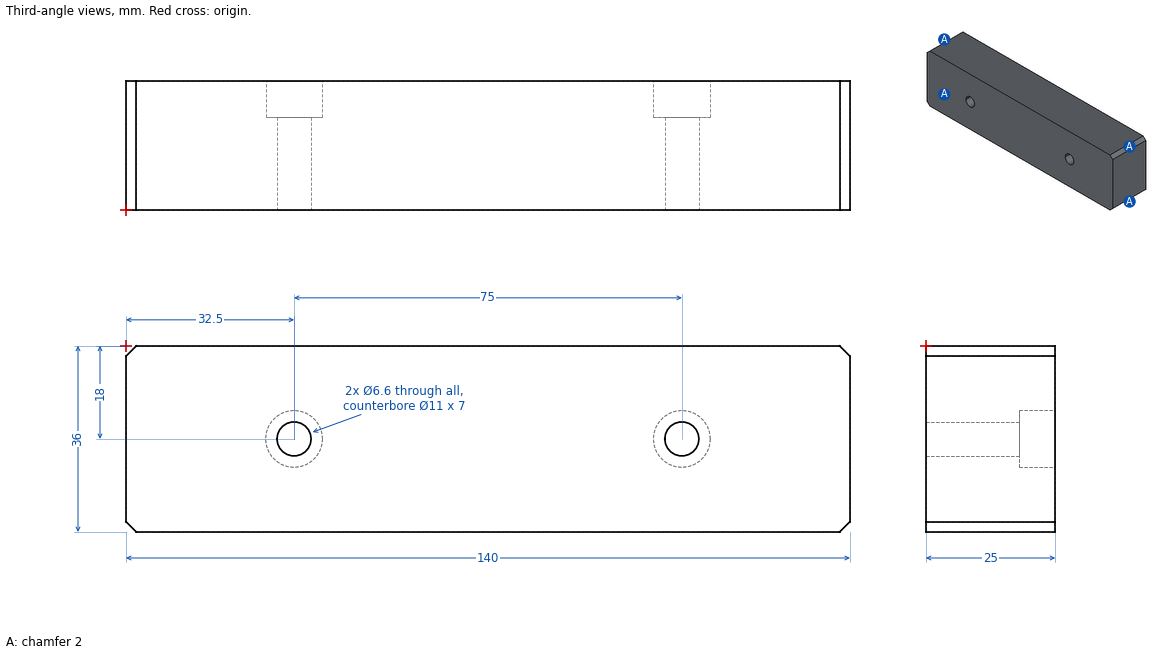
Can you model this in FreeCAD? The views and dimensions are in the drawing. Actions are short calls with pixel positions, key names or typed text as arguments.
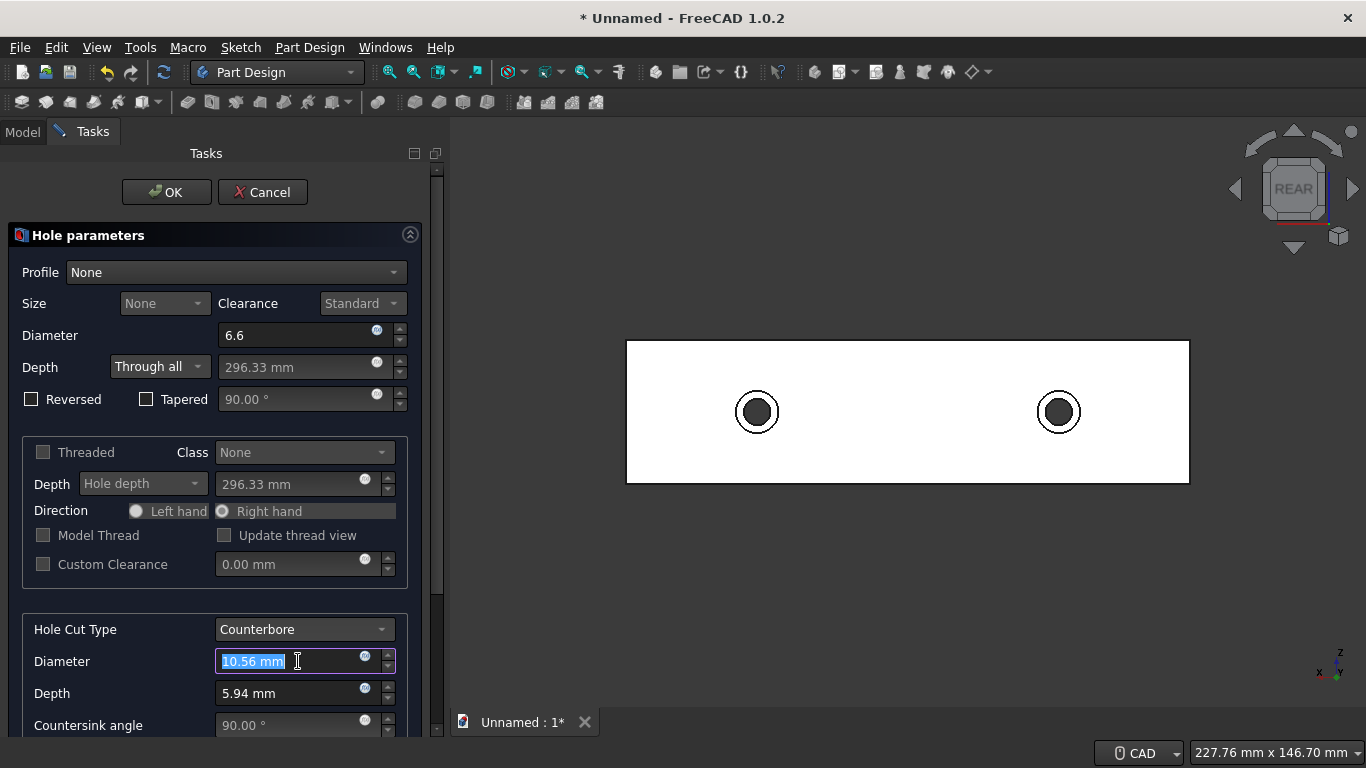
text(11)
key(Tab)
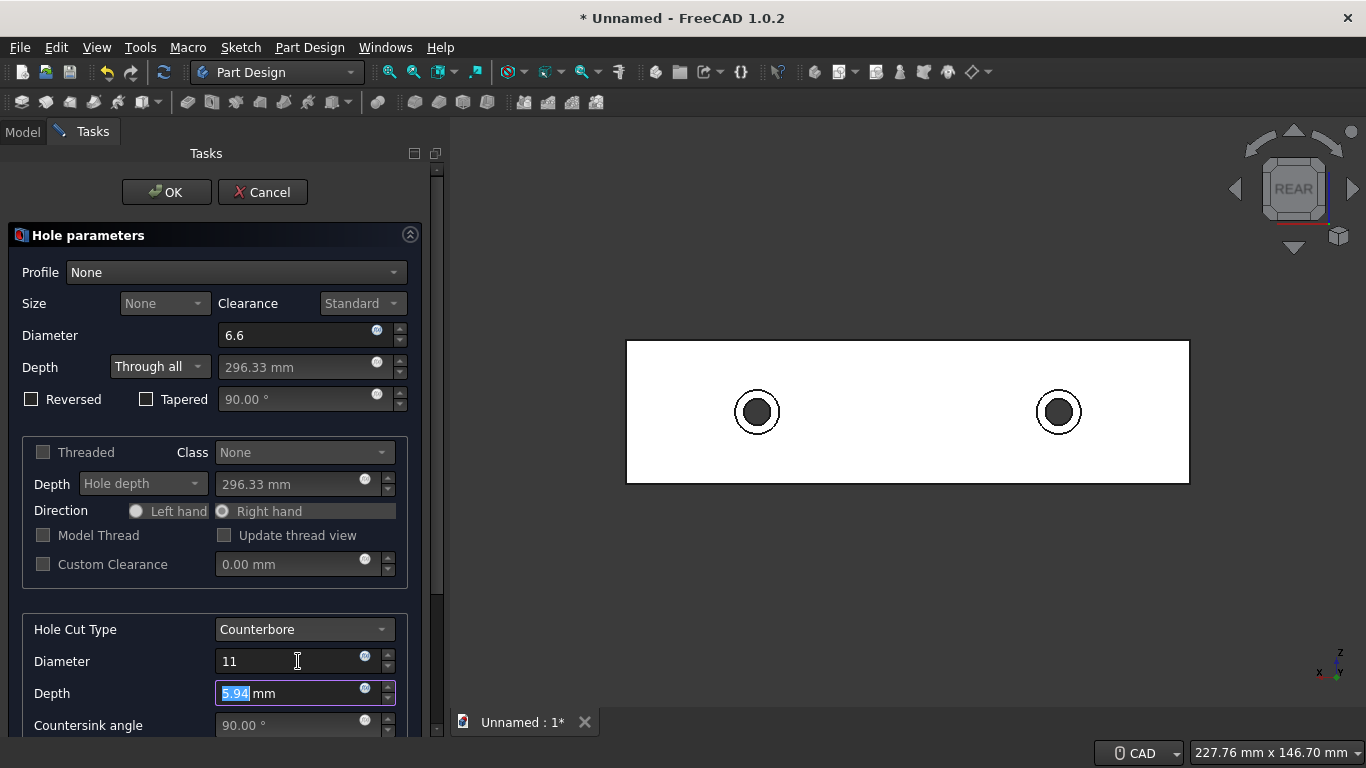
text(7)
key(Tab)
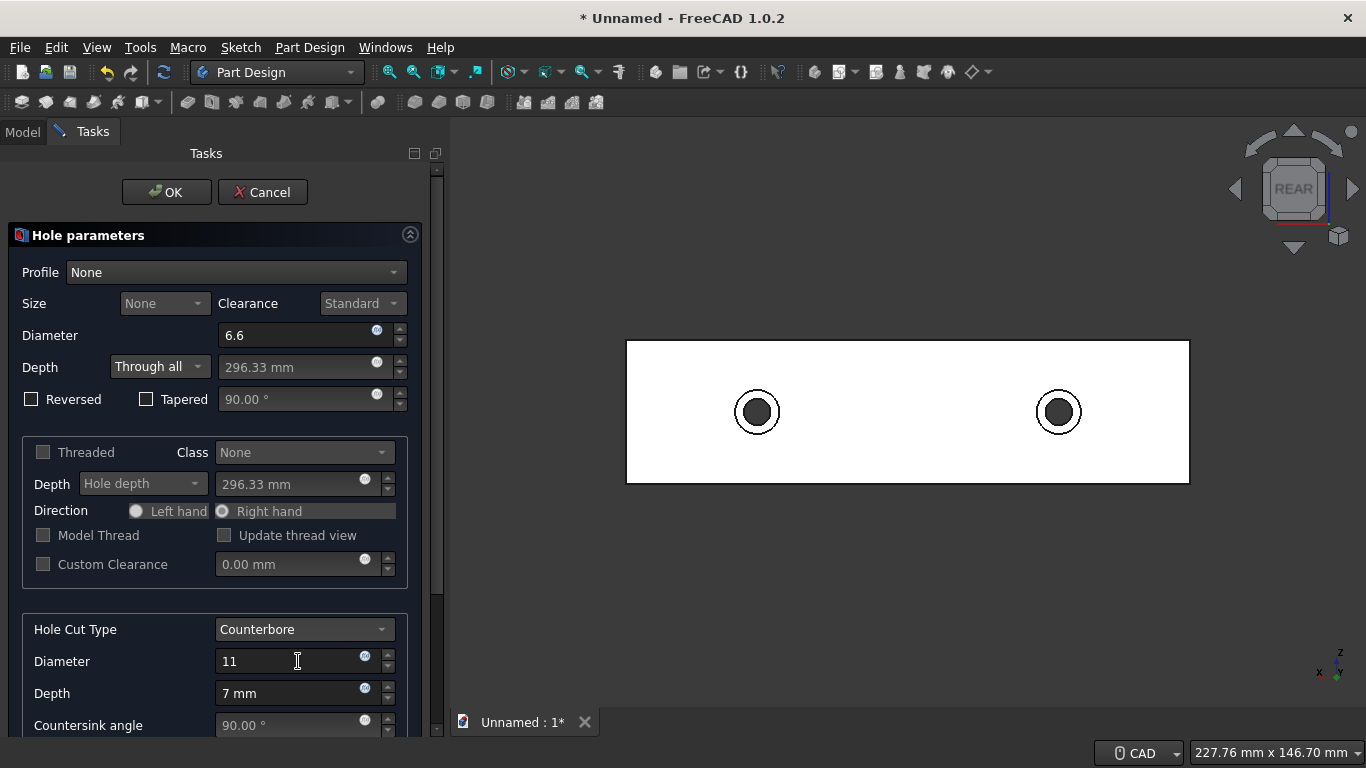
click(167, 192)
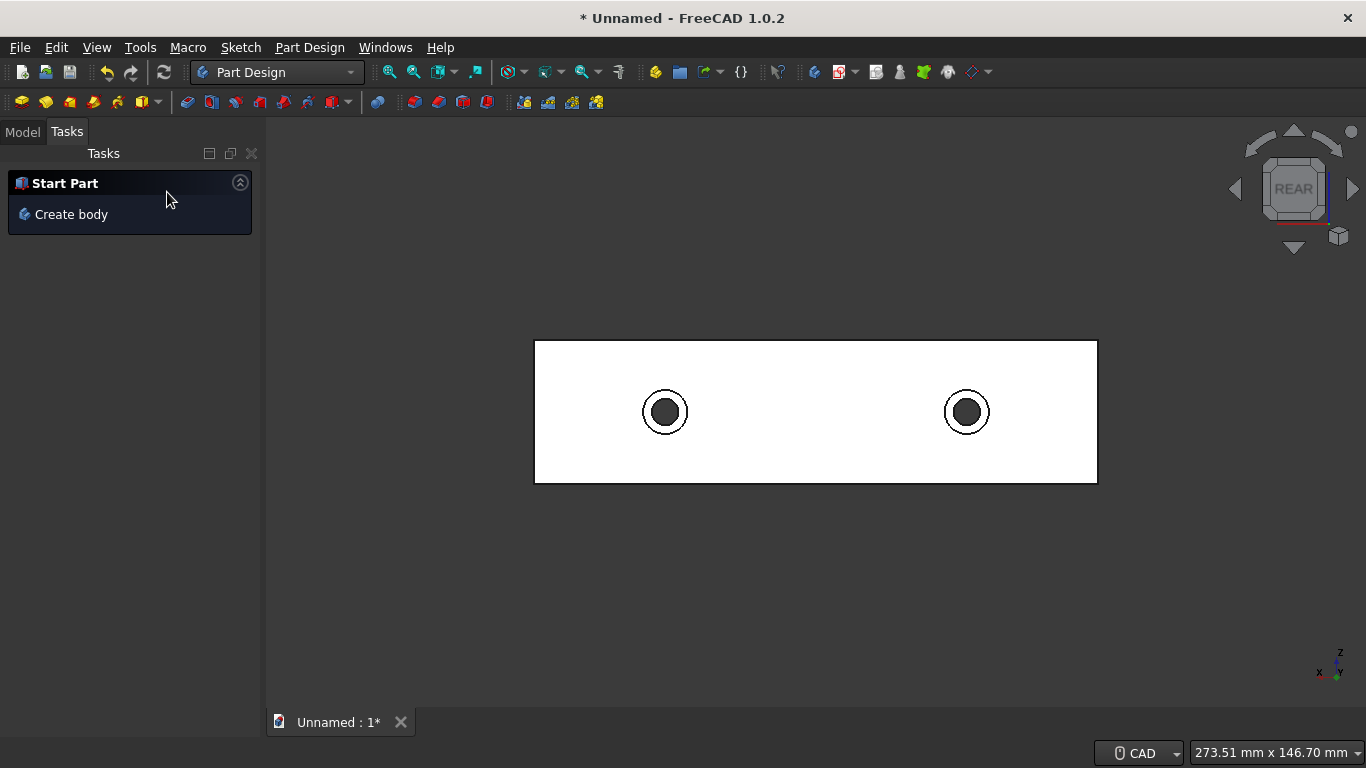
key(0)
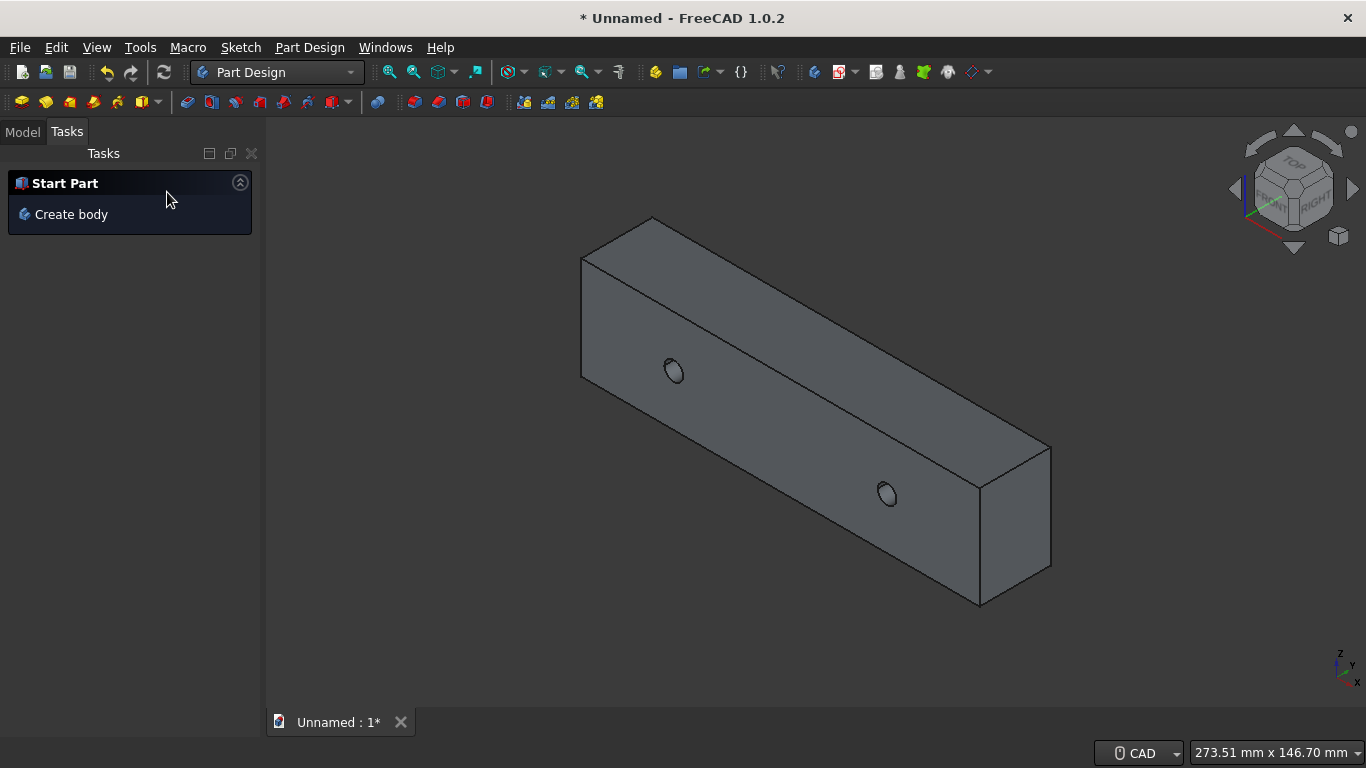
click(1015, 467)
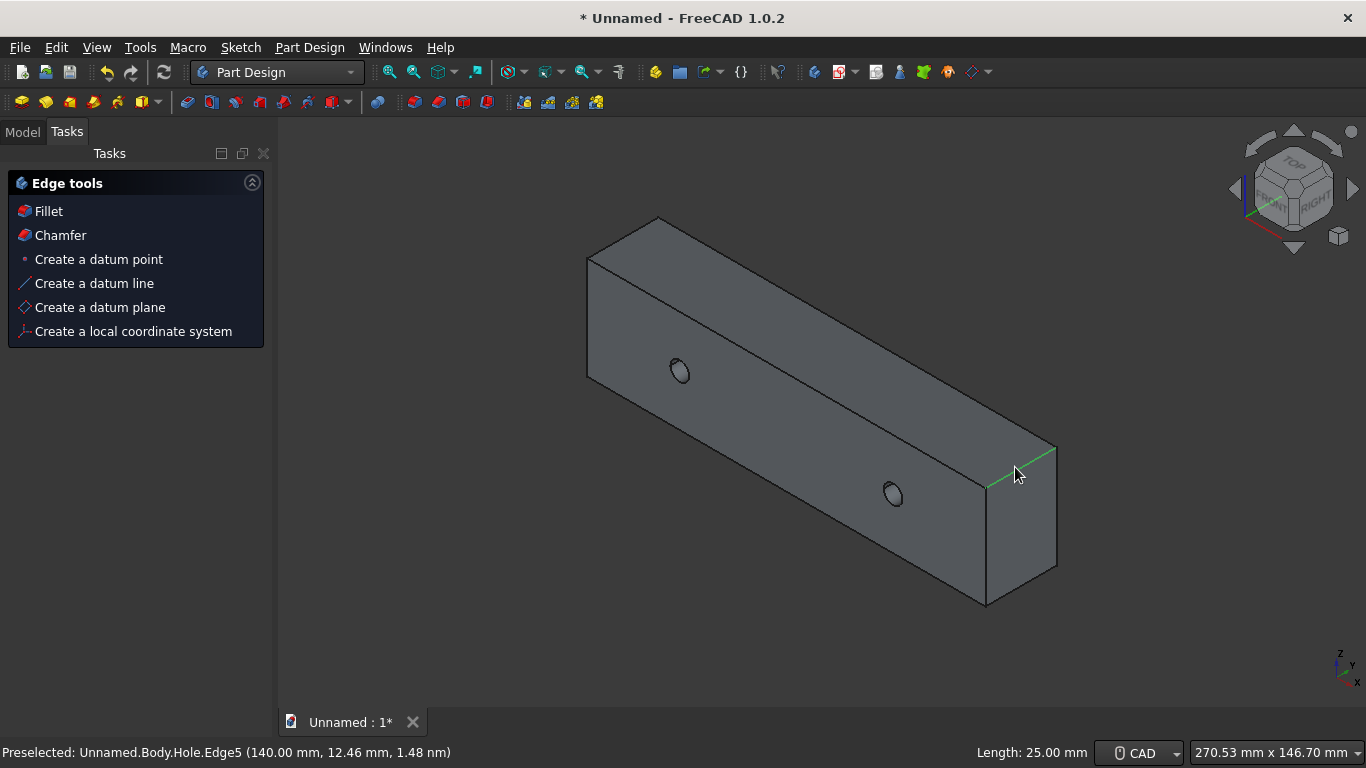
key(2)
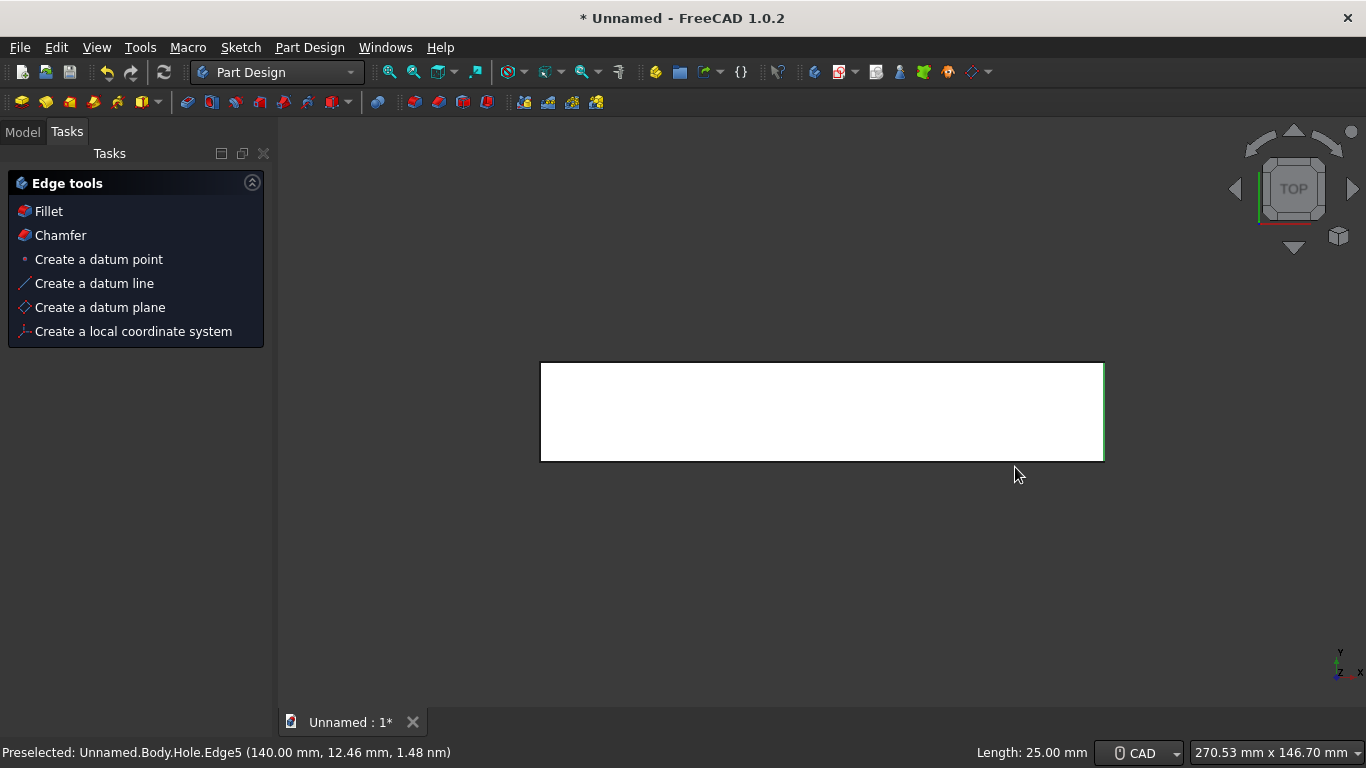
click(540, 421, ctrl)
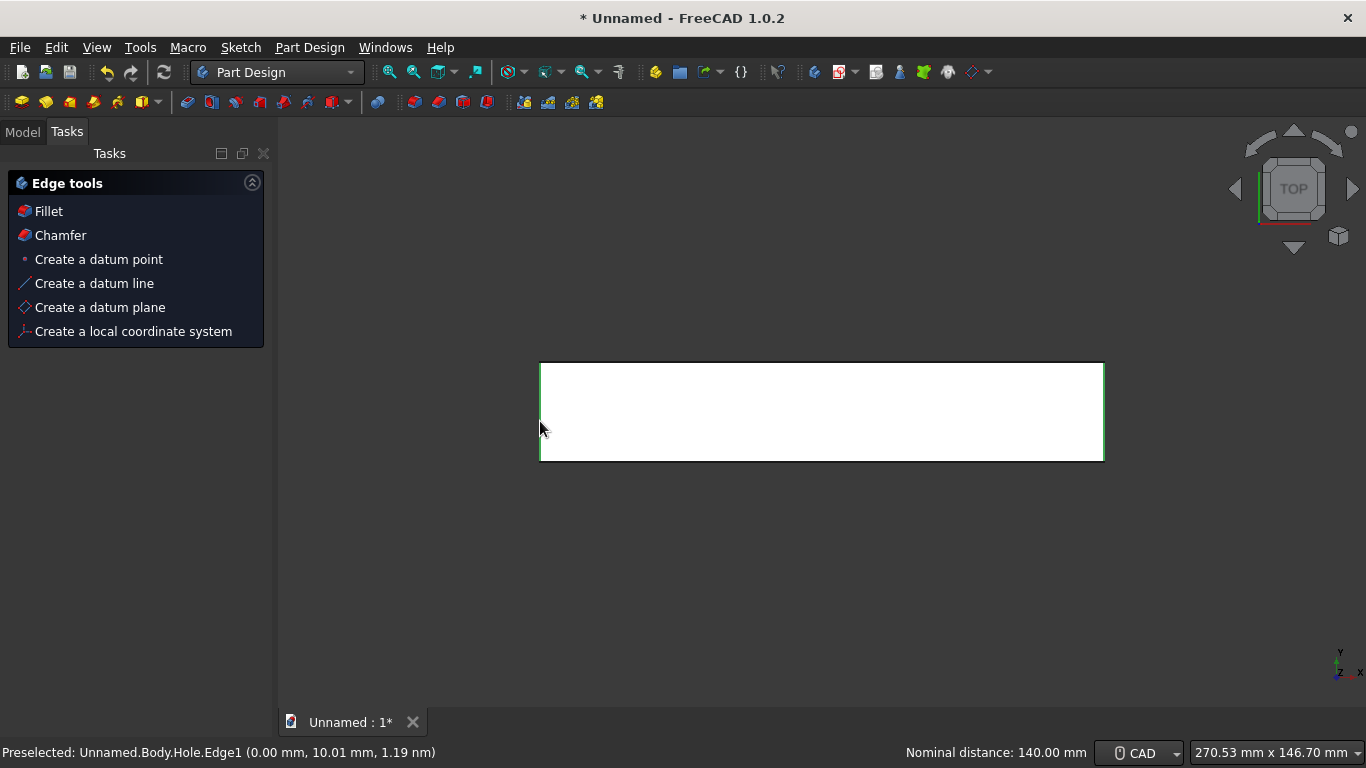
key(1)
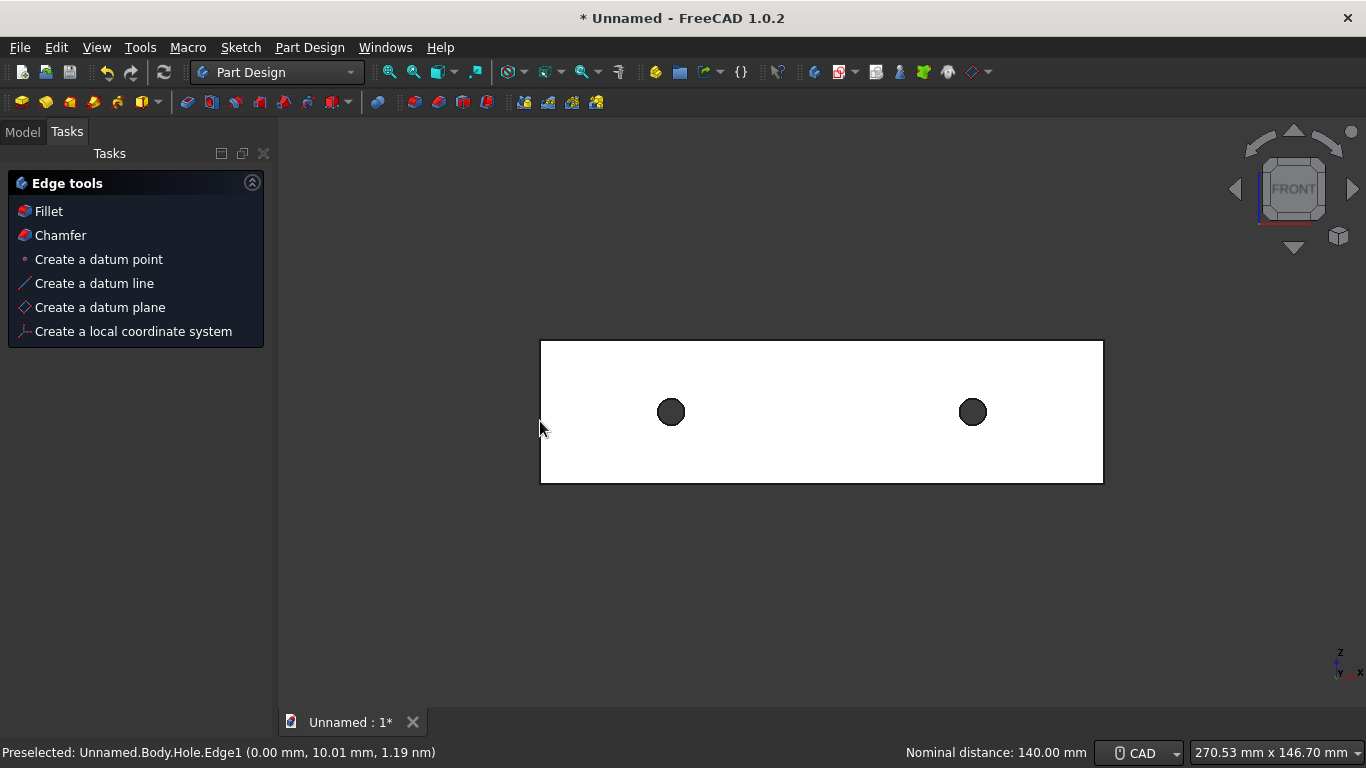
key(3)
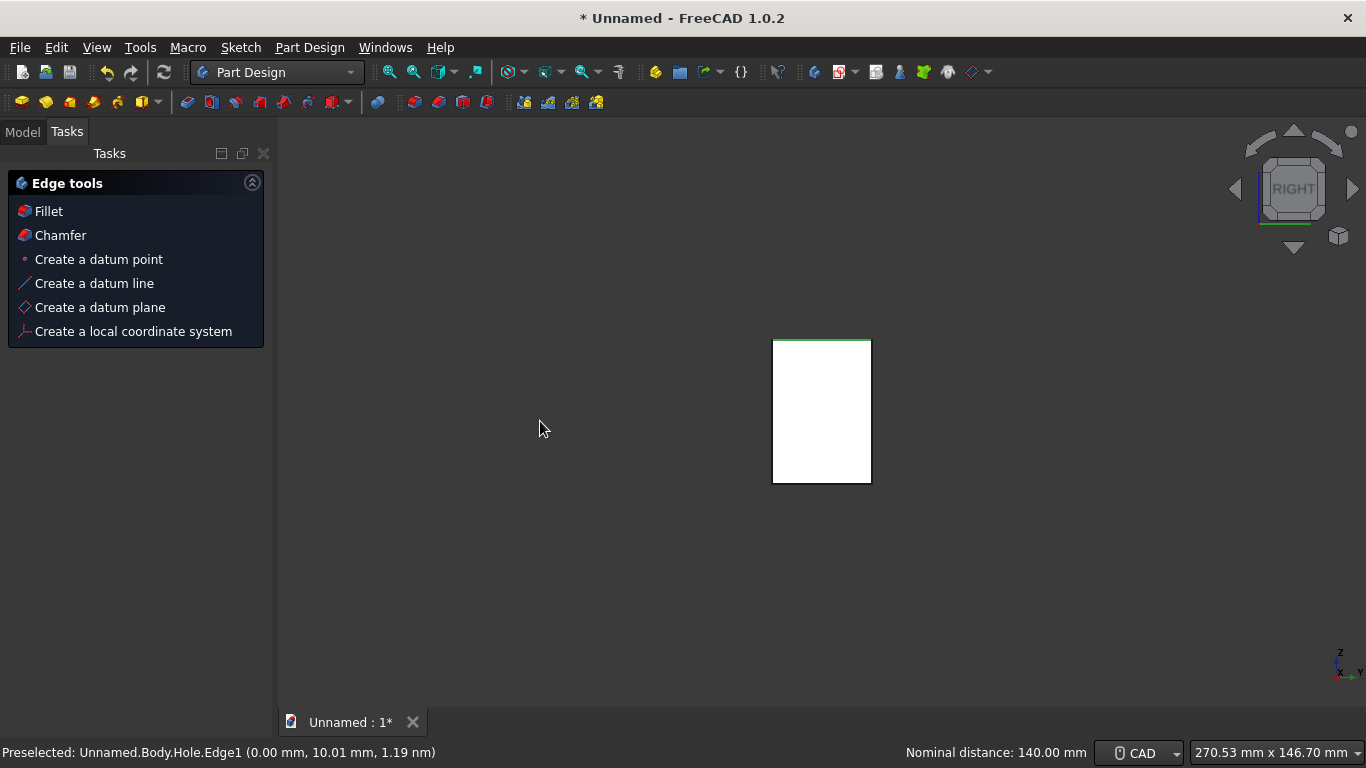
click(390, 72)